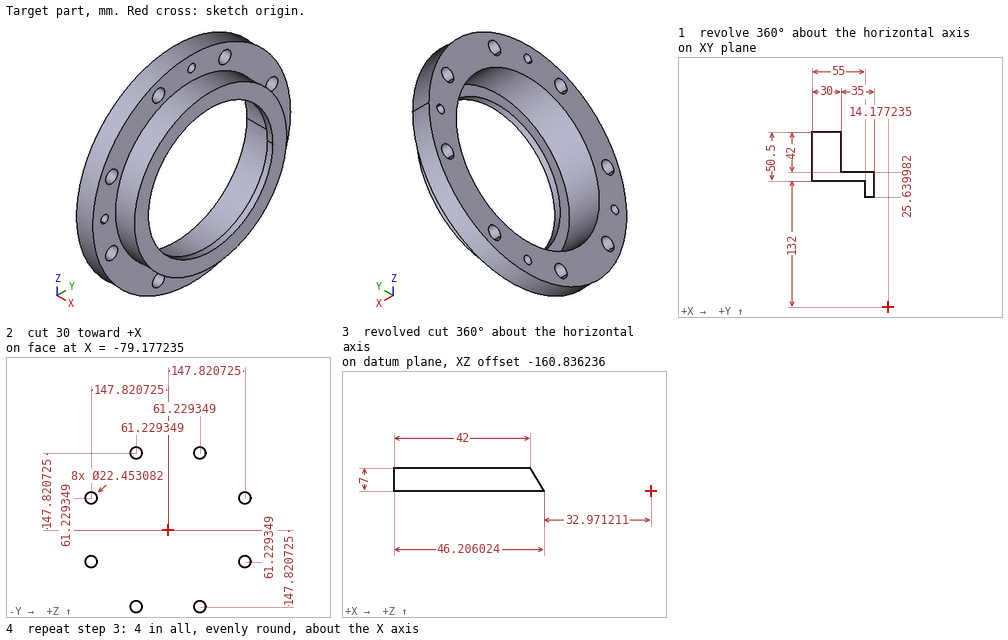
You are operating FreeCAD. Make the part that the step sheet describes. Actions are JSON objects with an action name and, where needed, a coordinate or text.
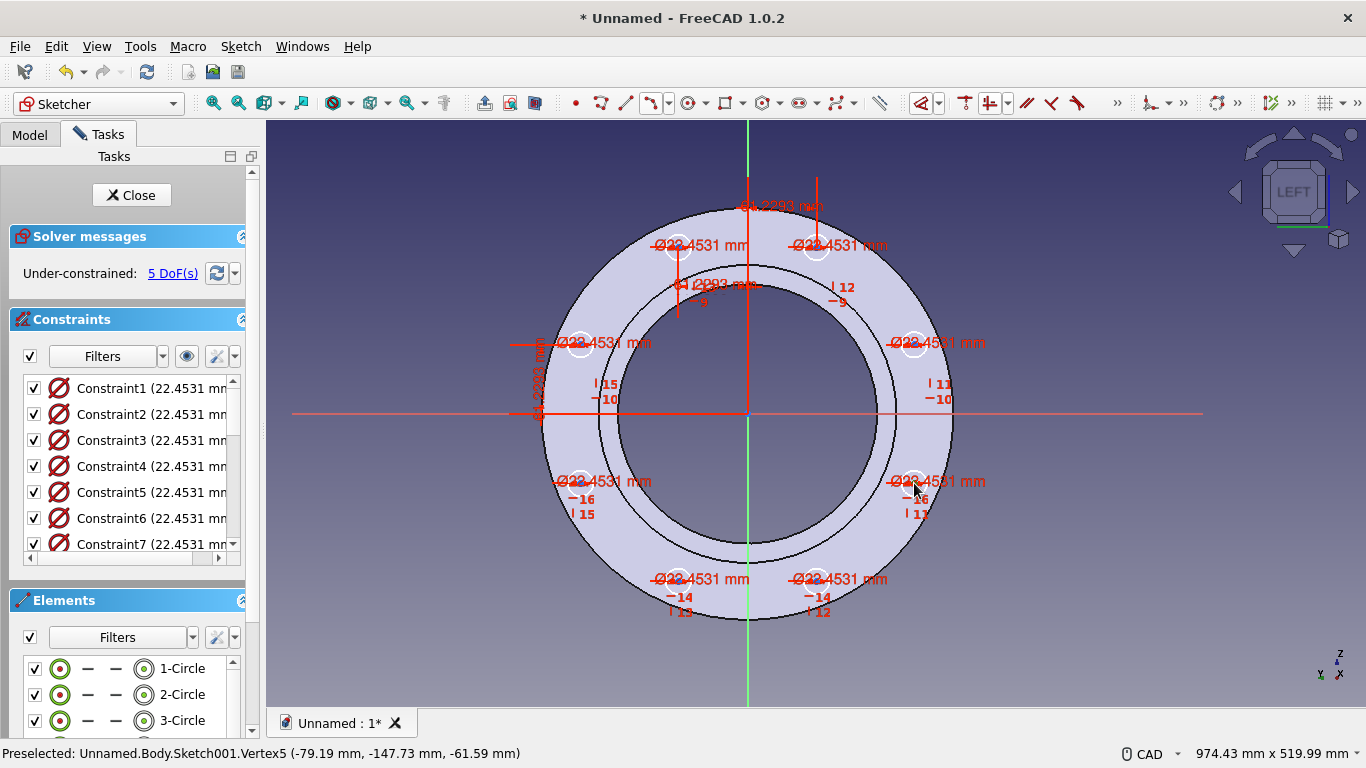
{"action": "left_click", "coordinate": [938, 104]}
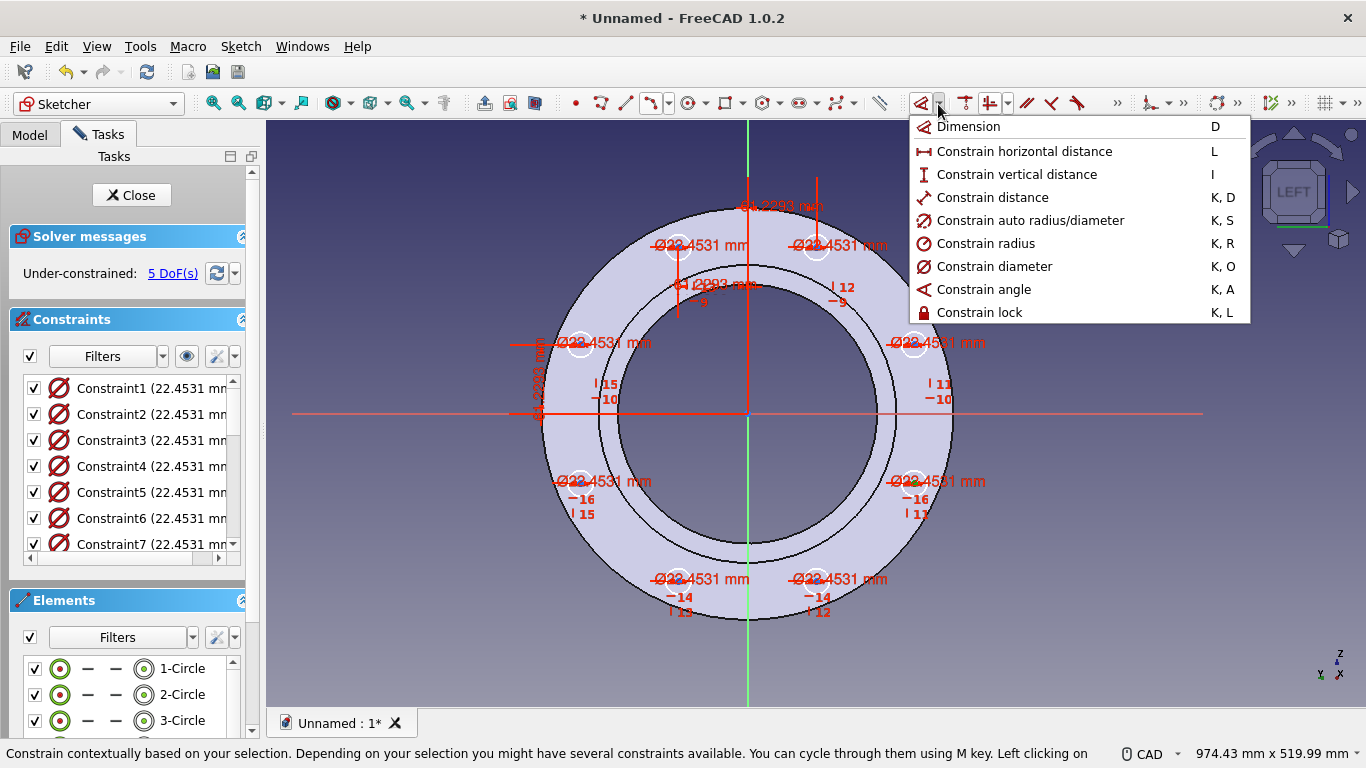
{"action": "left_click", "coordinate": [1080, 174]}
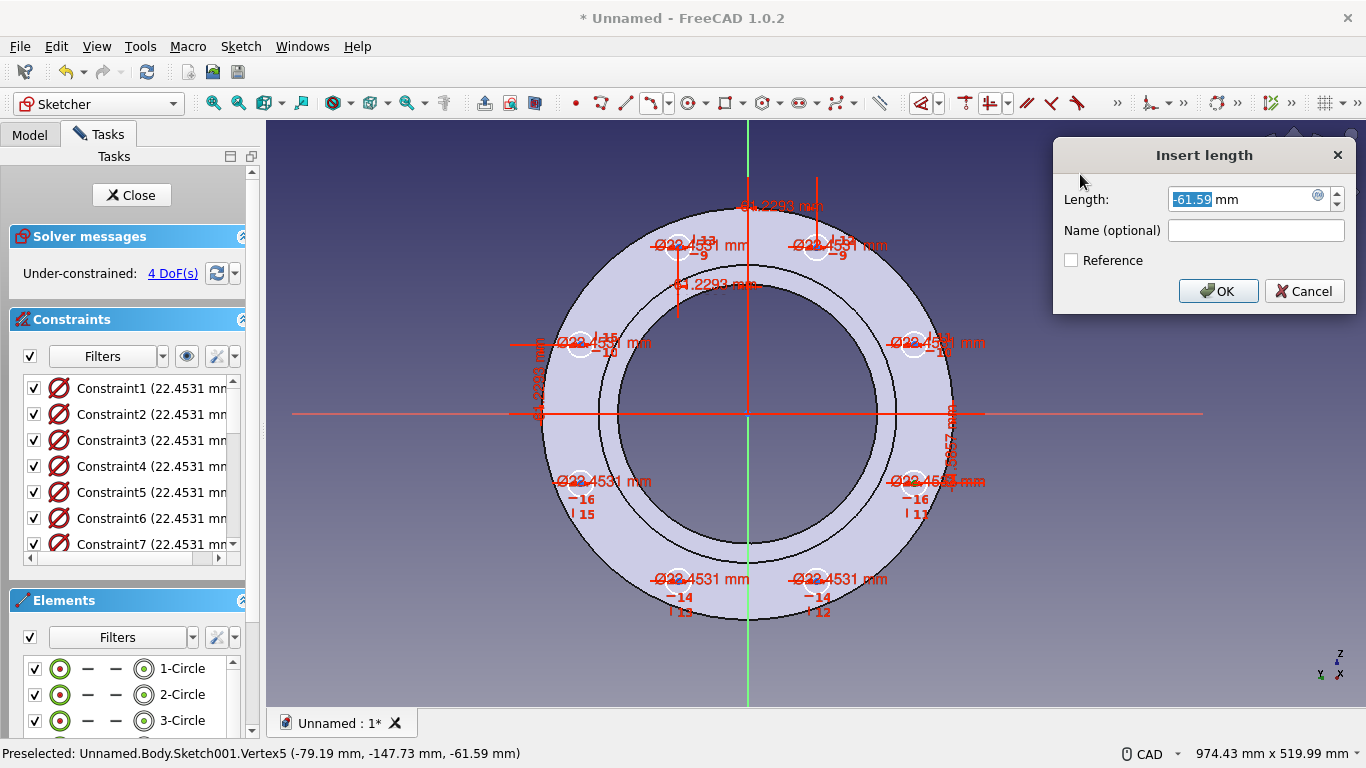
{"action": "type", "text": "-61.229349"}
{"action": "key", "text": "Return"}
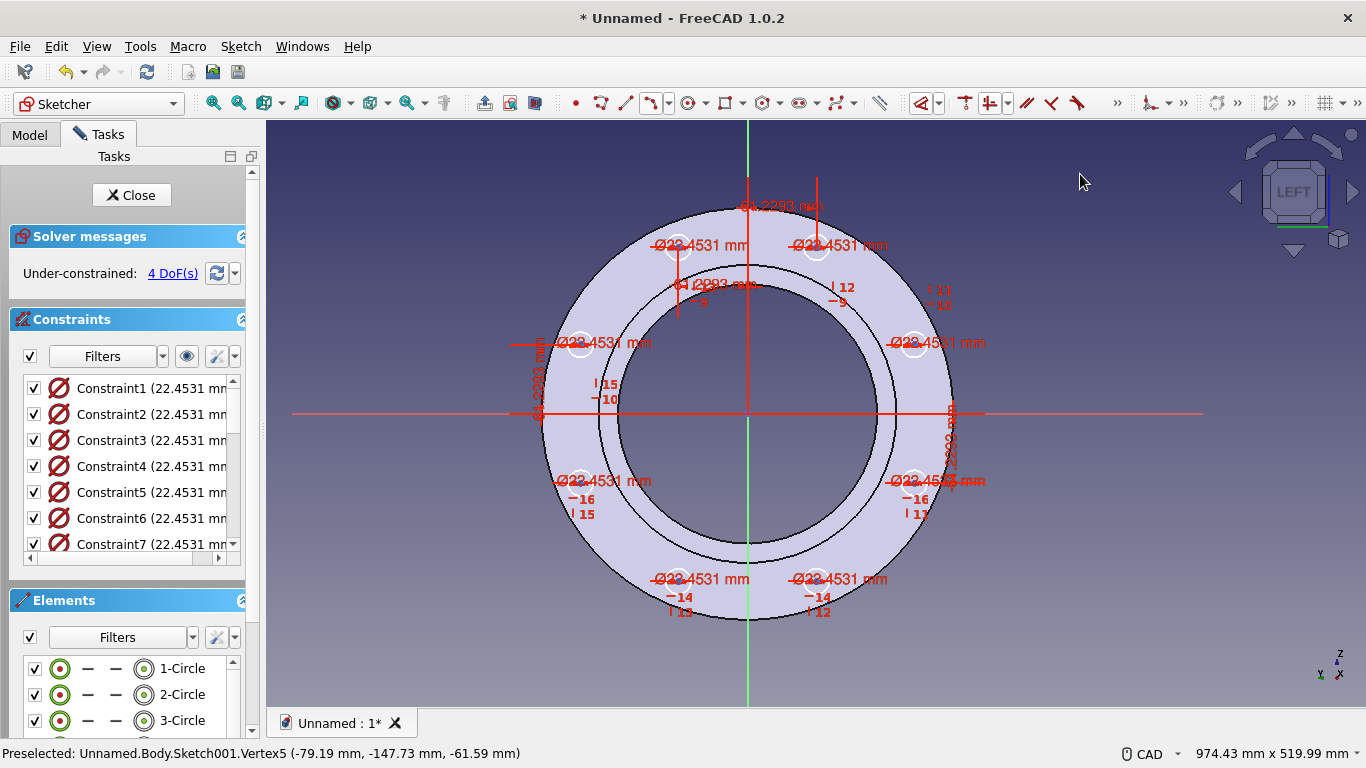
{"action": "left_click", "coordinate": [581, 345]}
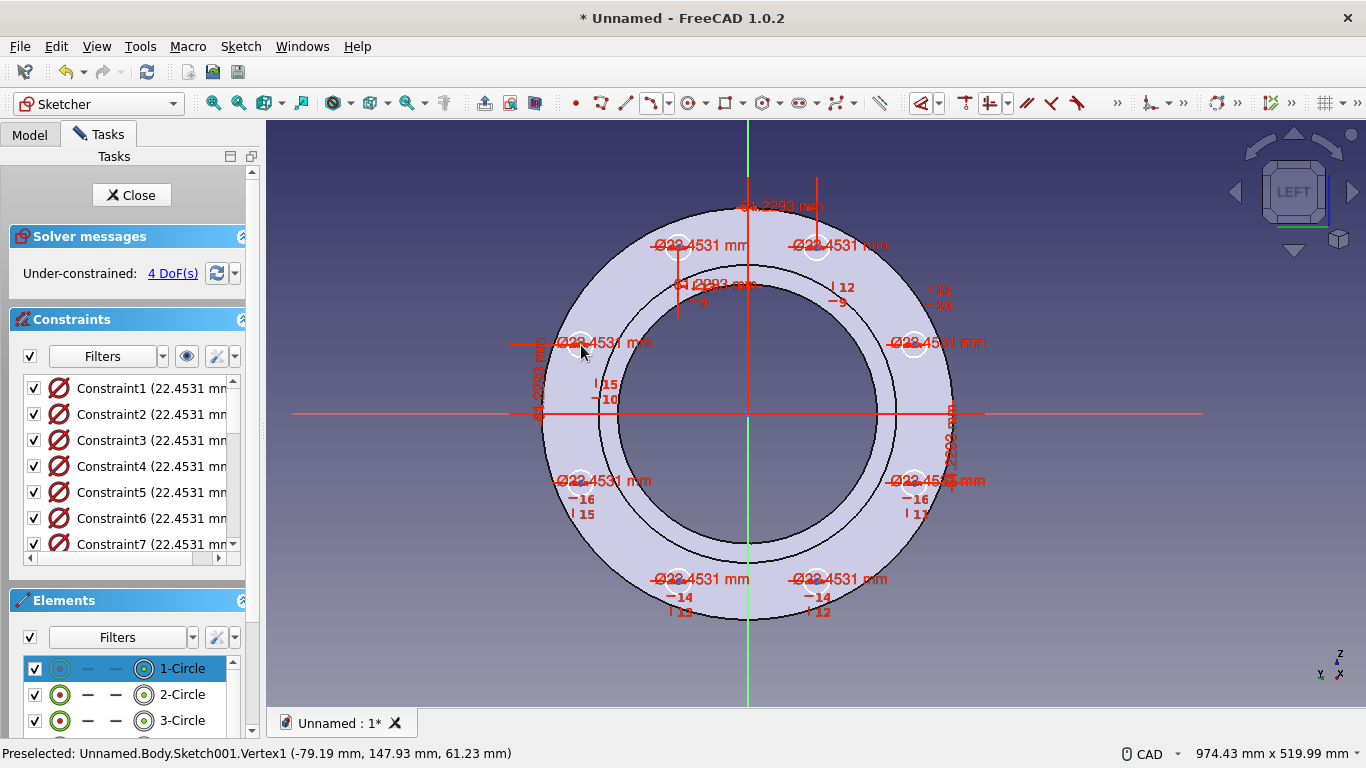
{"action": "left_click", "coordinate": [938, 104]}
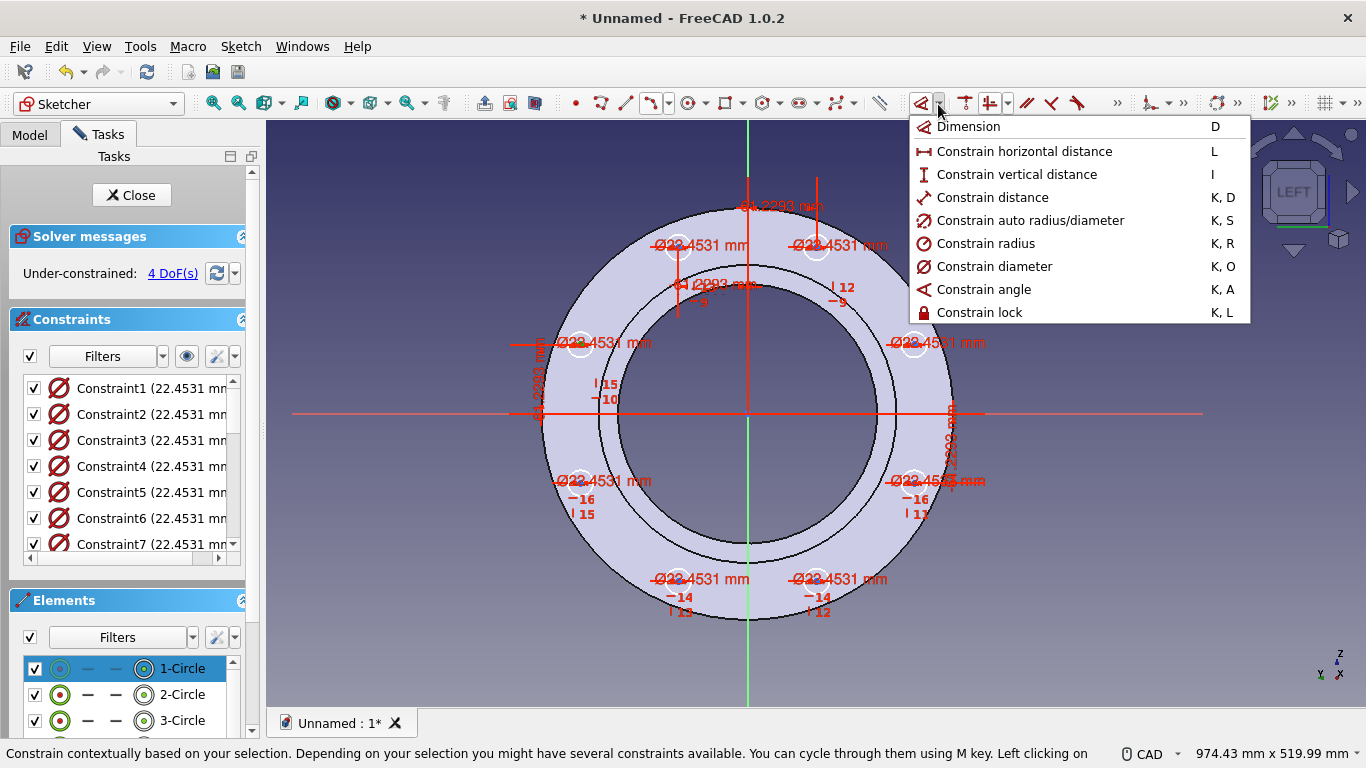
{"action": "left_click", "coordinate": [1080, 152]}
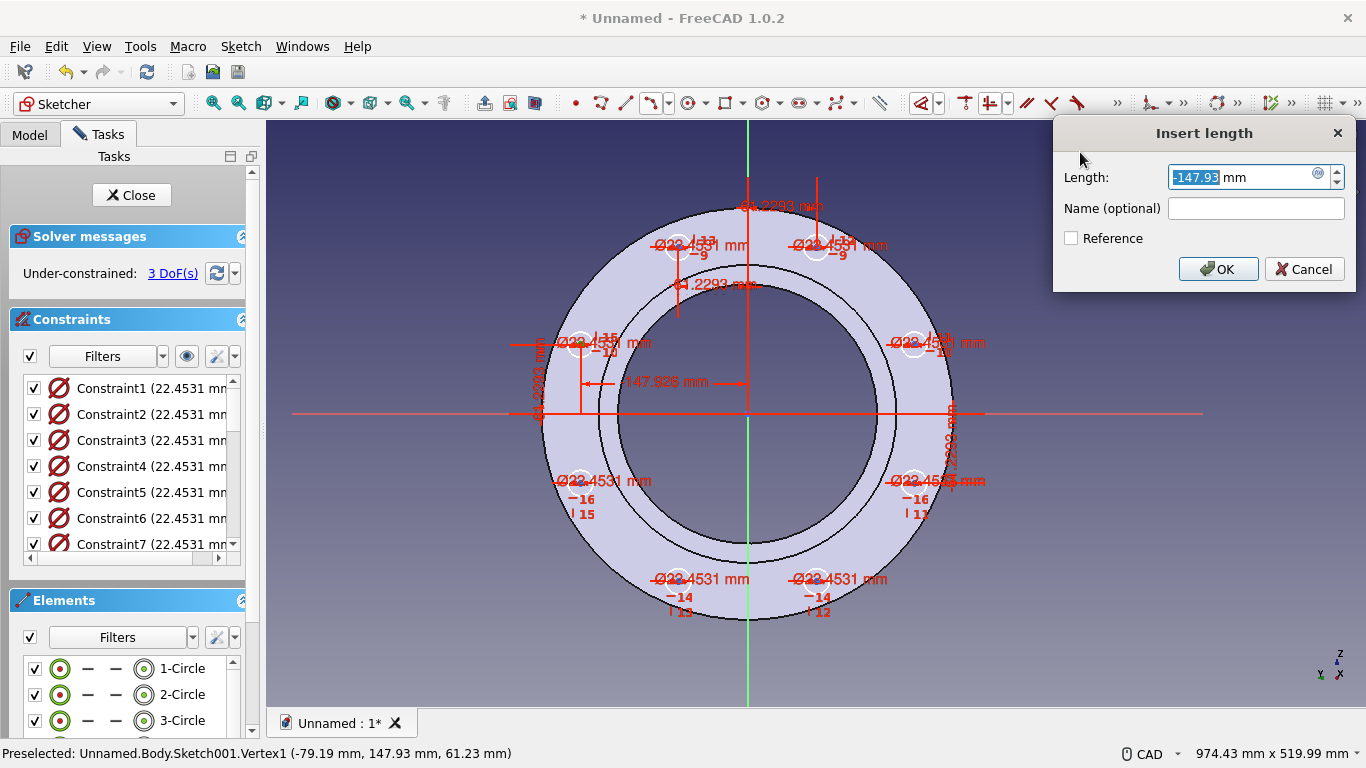
{"action": "type", "text": "-147.820725"}
{"action": "key", "text": "Return"}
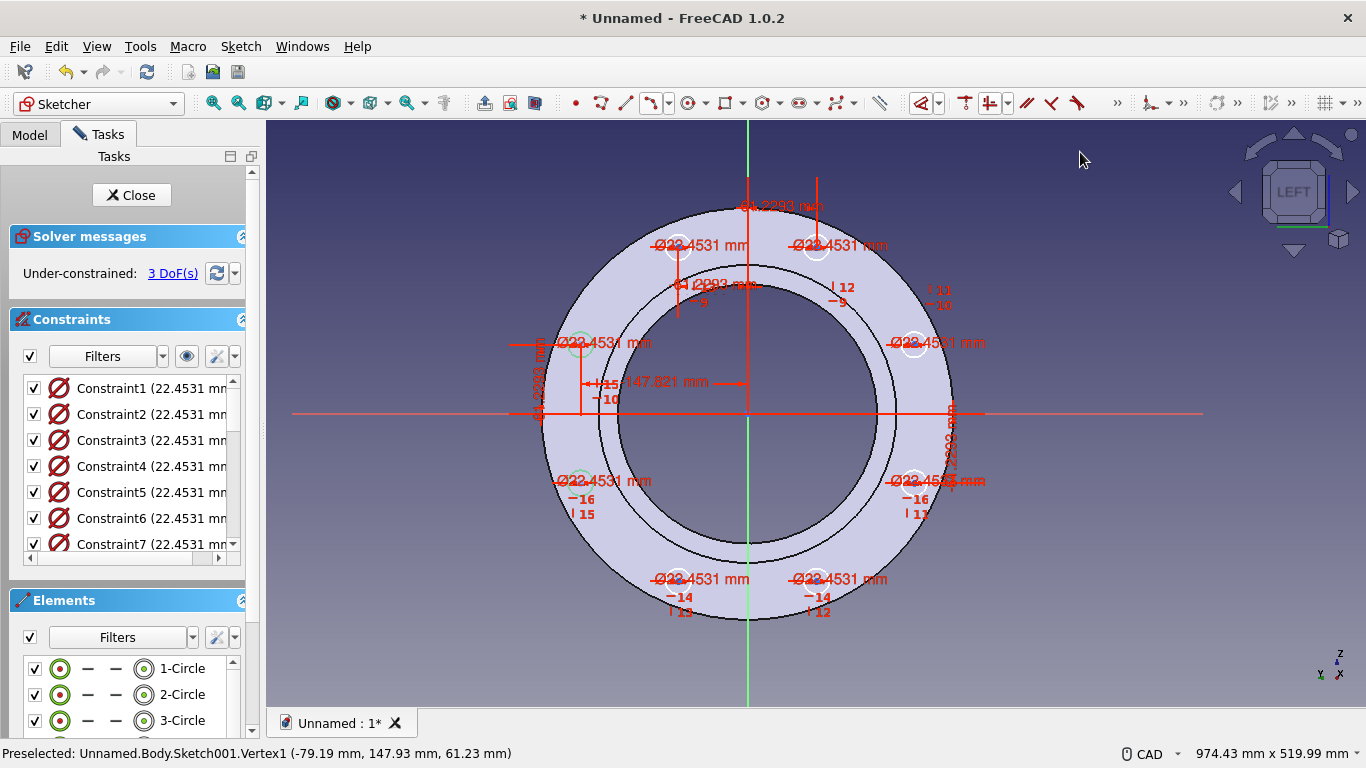
{"action": "left_click", "coordinate": [678, 247]}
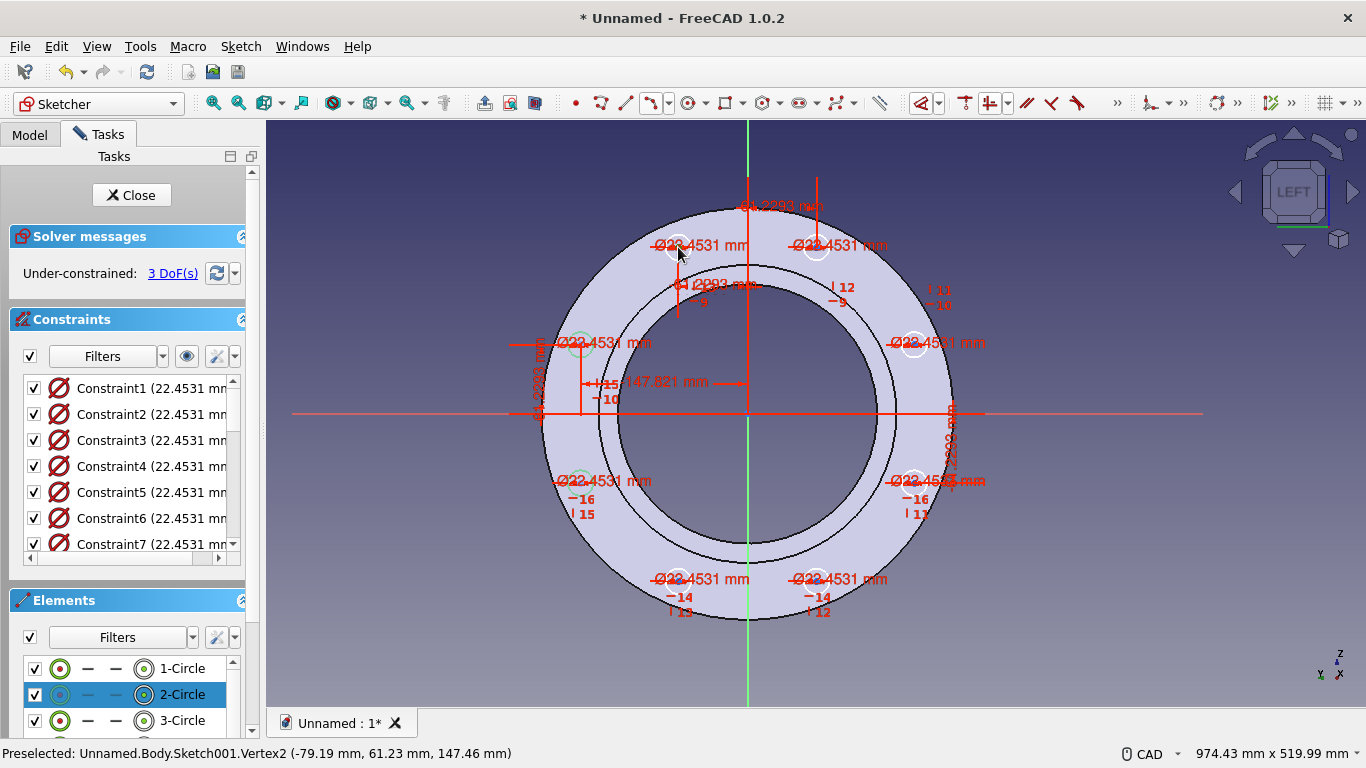
{"action": "key", "text": "i"}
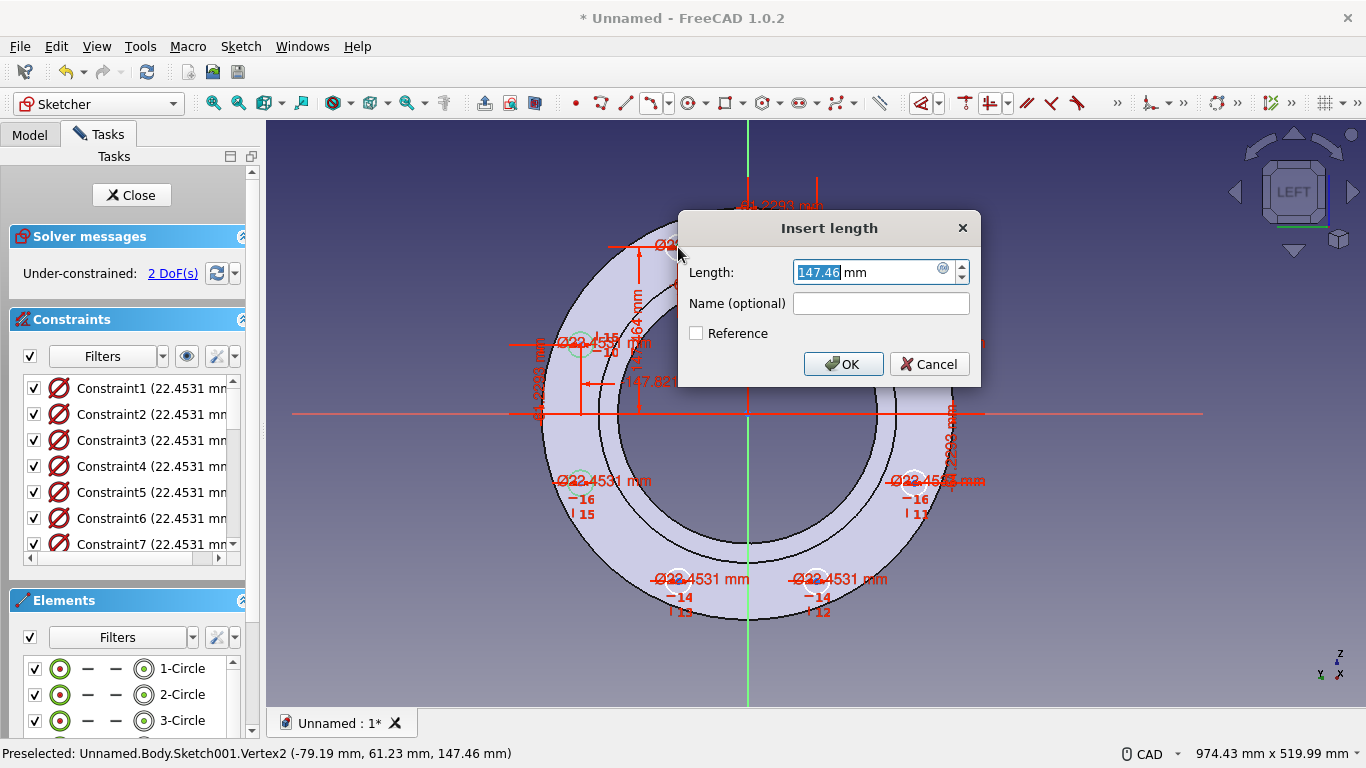
{"action": "type", "text": "147.820725"}
{"action": "key", "text": "Return"}